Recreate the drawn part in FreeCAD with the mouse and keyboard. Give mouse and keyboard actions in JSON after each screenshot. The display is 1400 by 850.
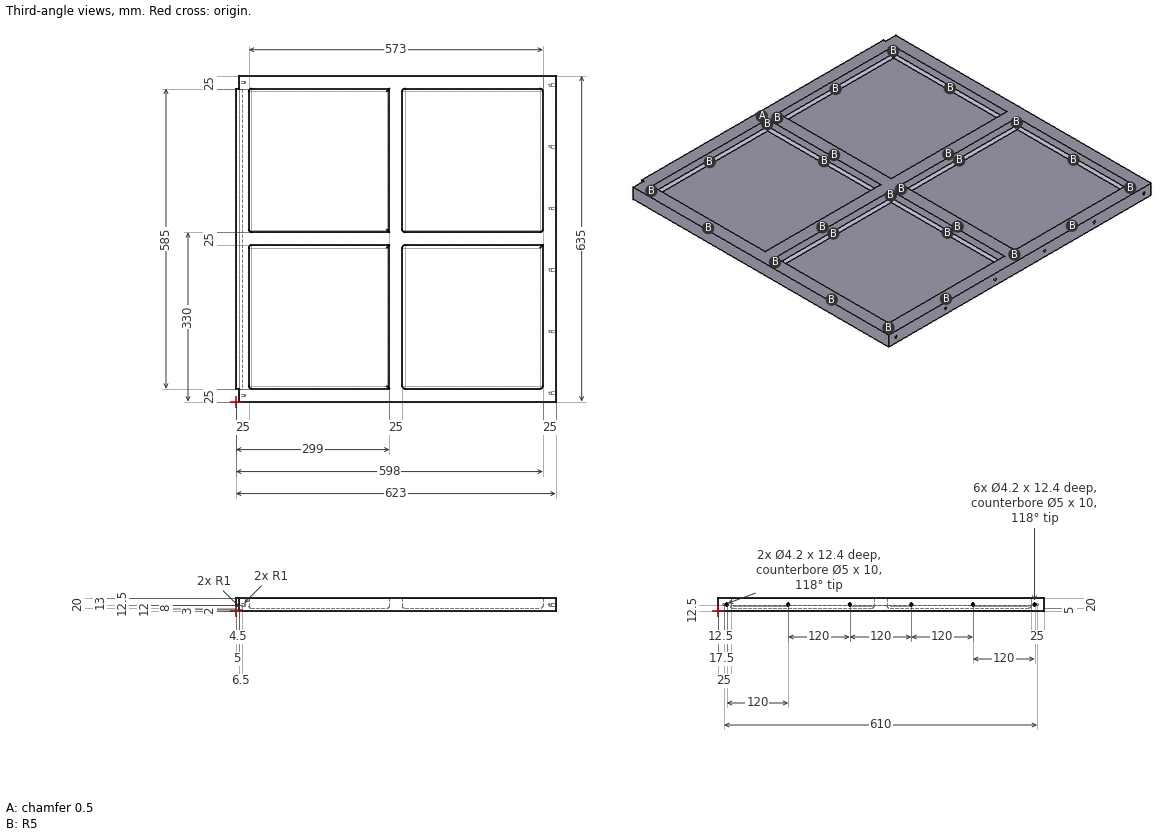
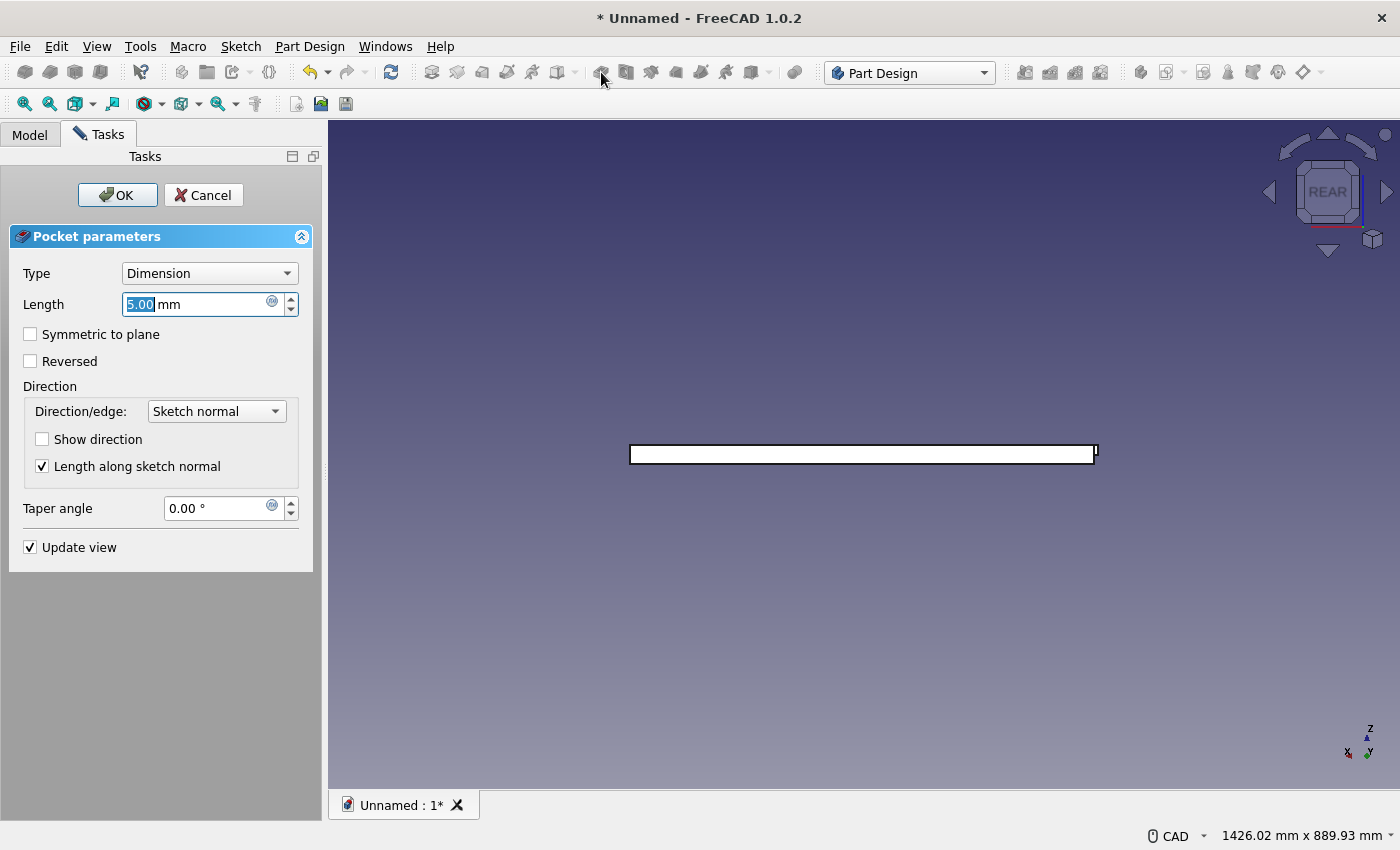
{"action": "type", "text": "25"}
{"action": "key", "text": "Tab"}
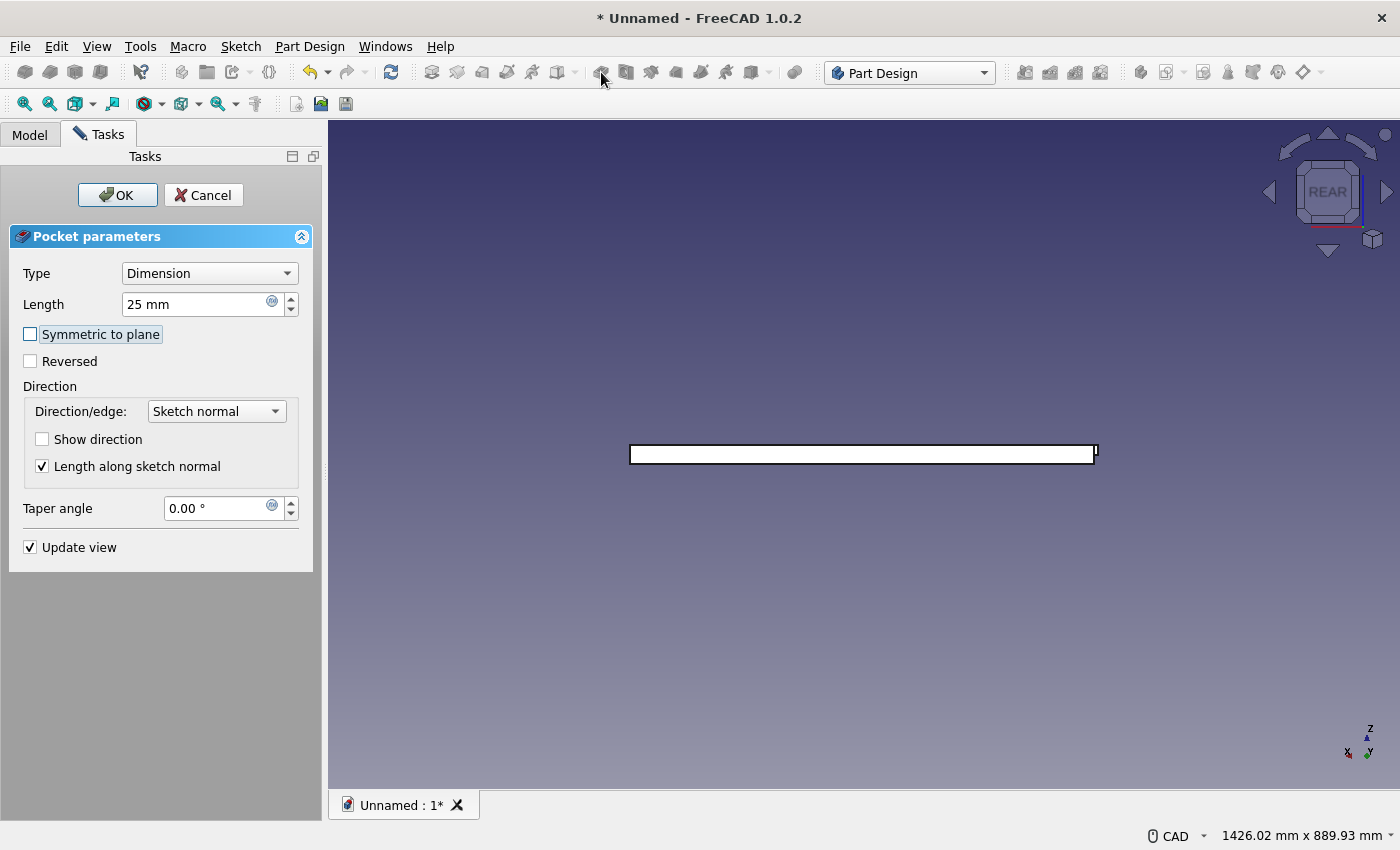
{"action": "left_click", "coordinate": [118, 195]}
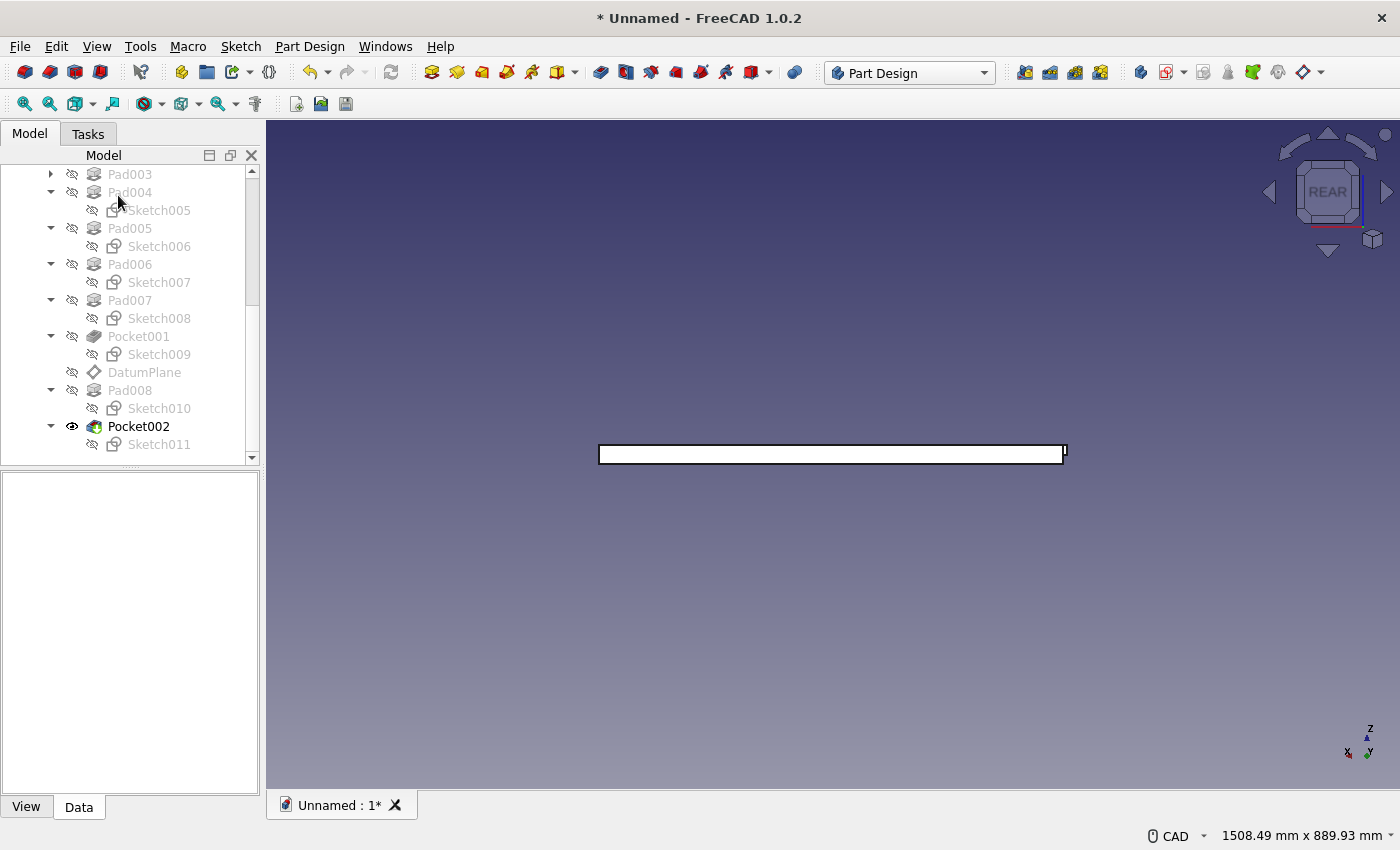
{"action": "left_click", "coordinate": [25, 104]}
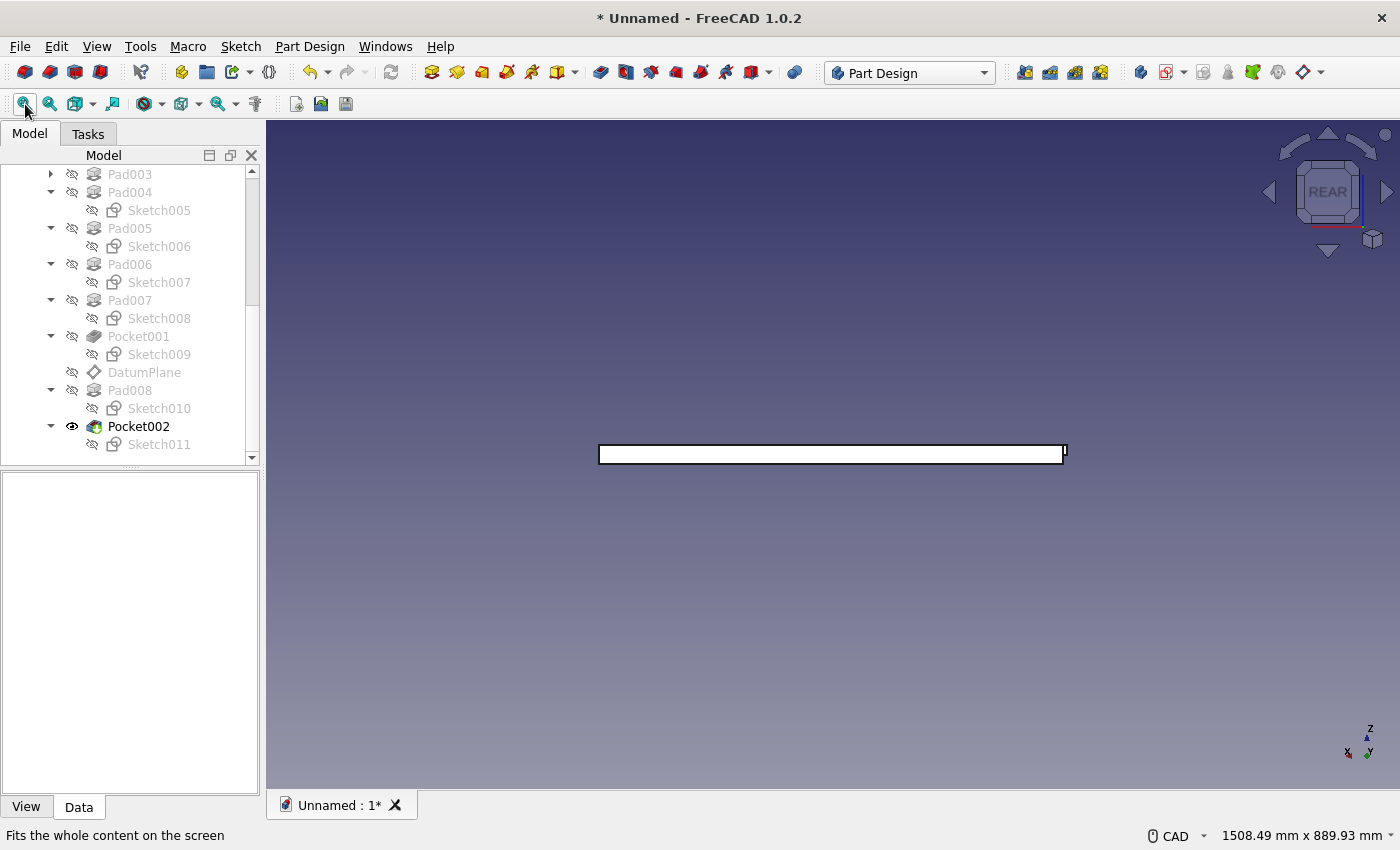
{"action": "key", "text": "0"}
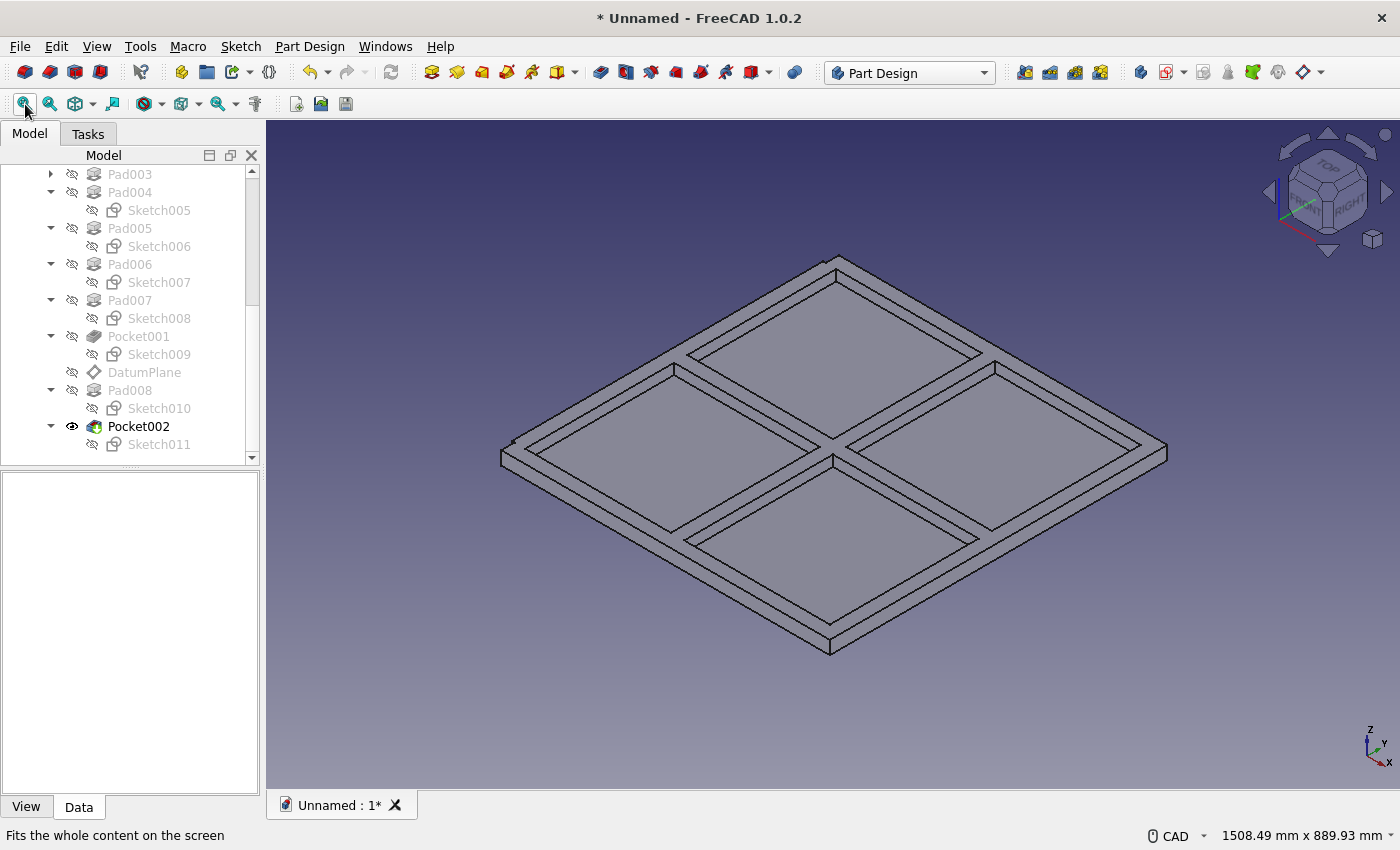
{"action": "key", "text": "3"}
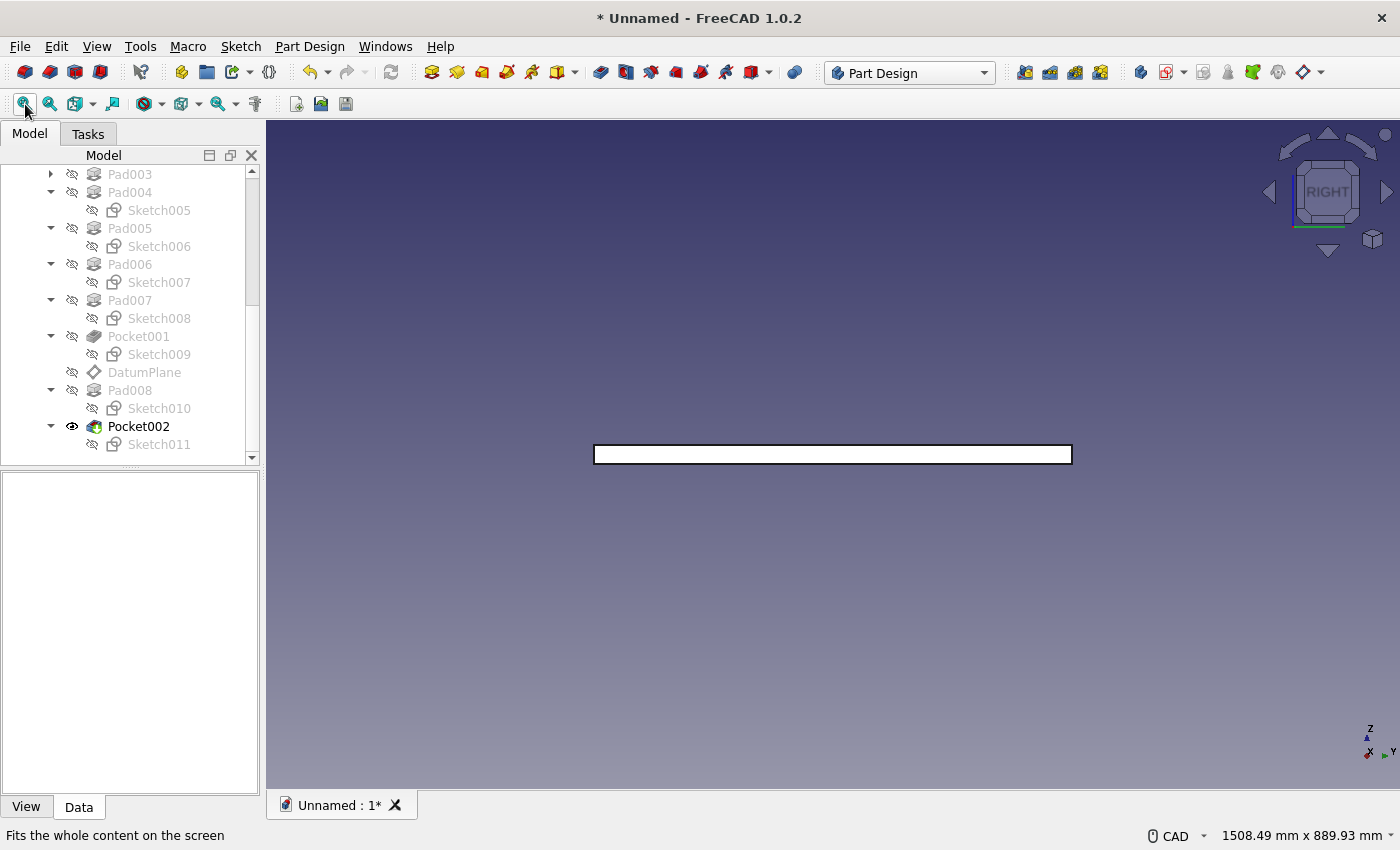
{"action": "key", "text": "v f"}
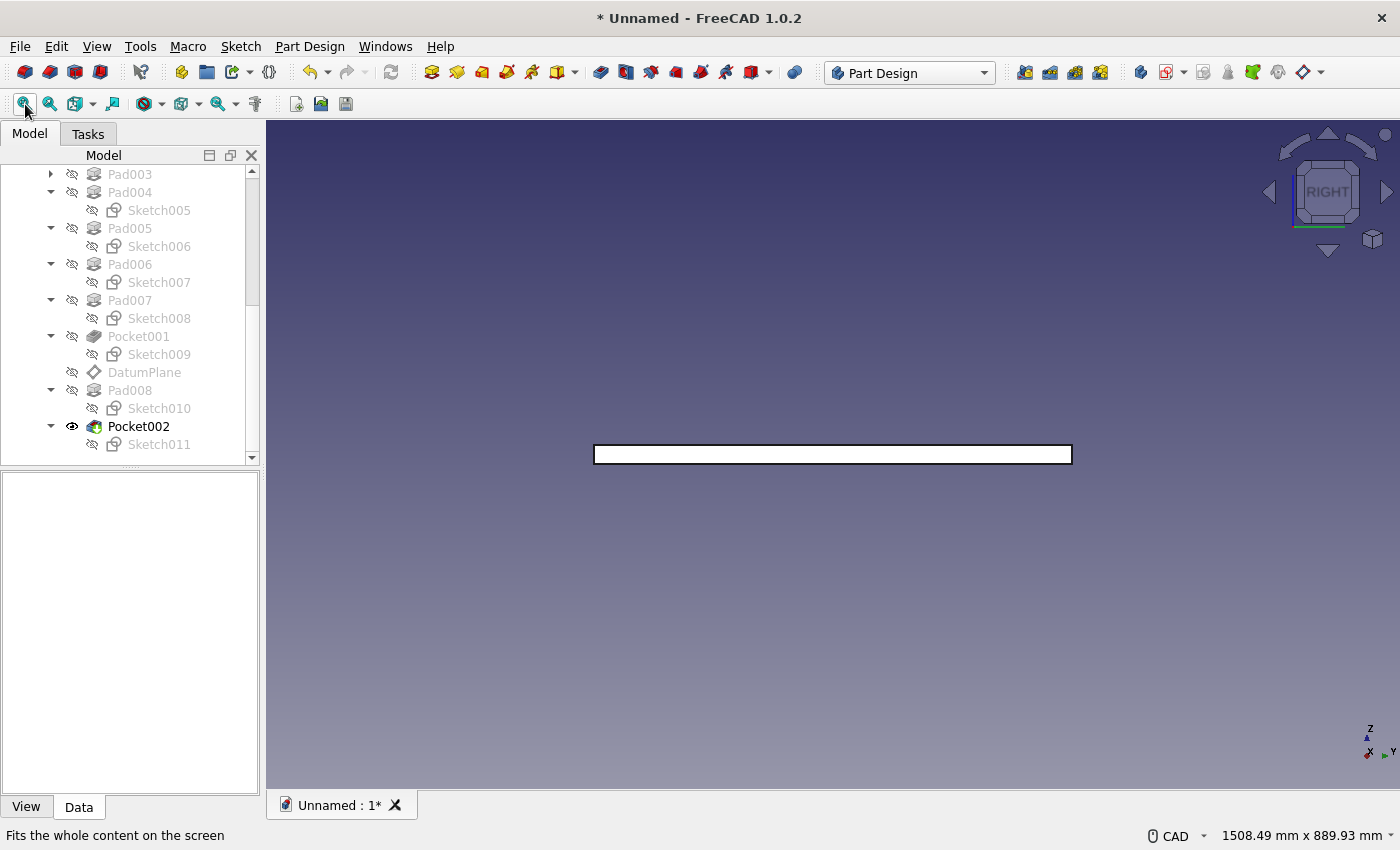
{"action": "left_click", "coordinate": [1038, 453]}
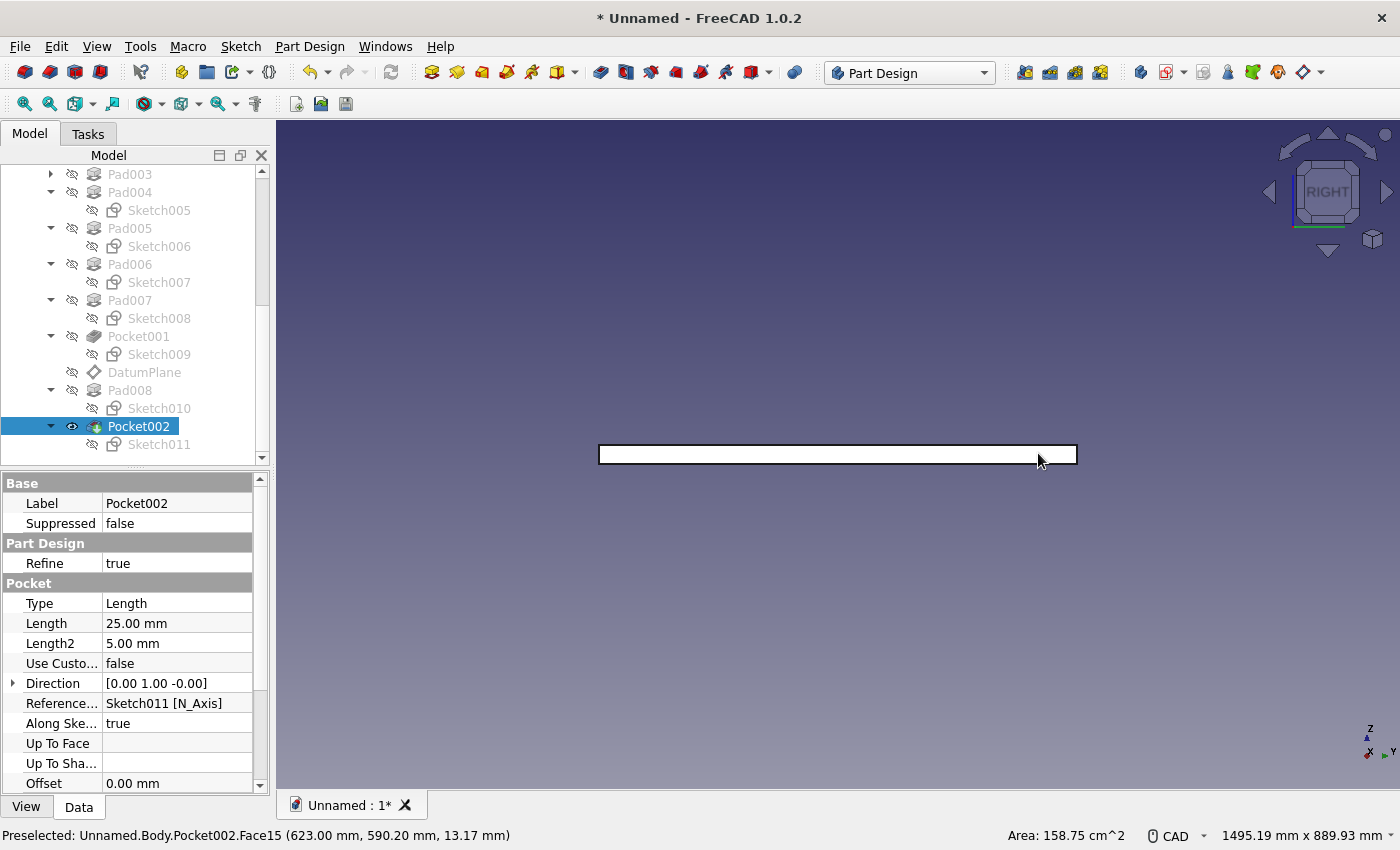
{"action": "left_click", "coordinate": [1166, 72]}